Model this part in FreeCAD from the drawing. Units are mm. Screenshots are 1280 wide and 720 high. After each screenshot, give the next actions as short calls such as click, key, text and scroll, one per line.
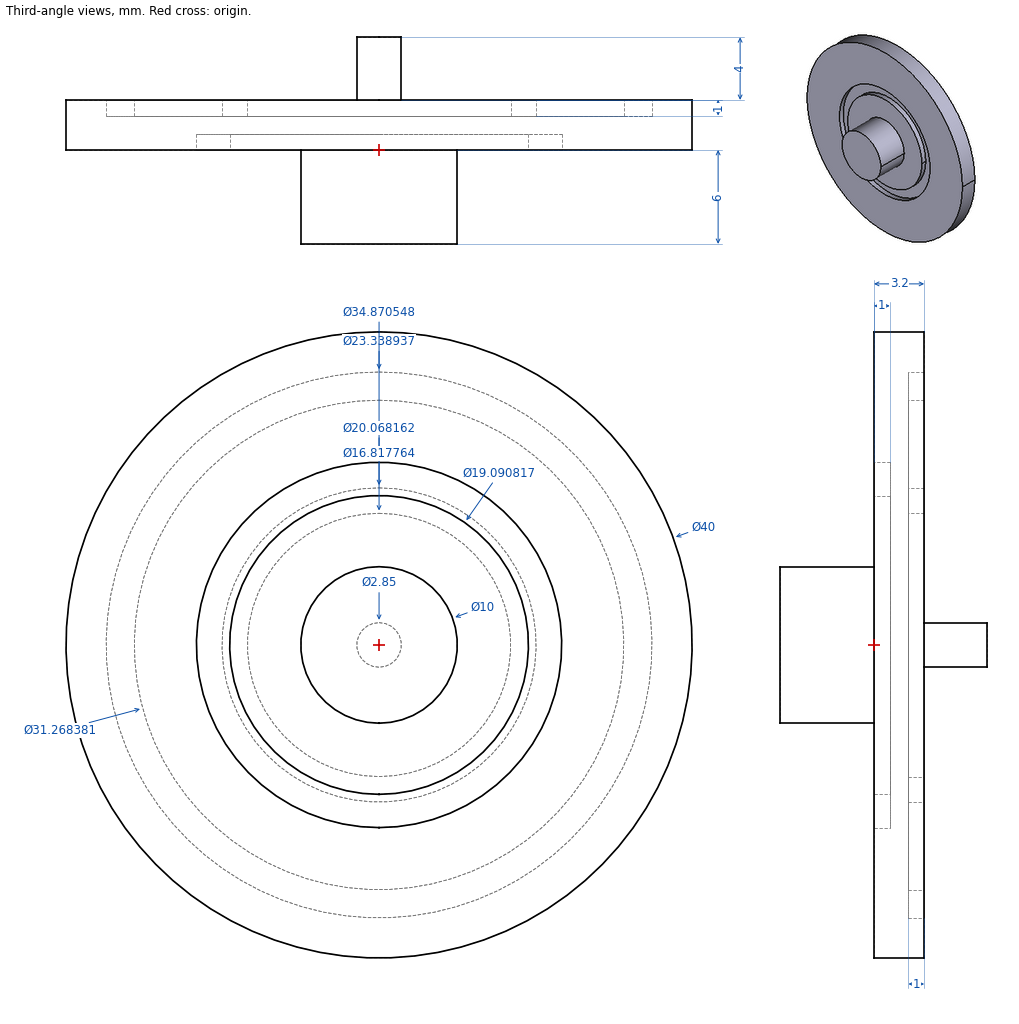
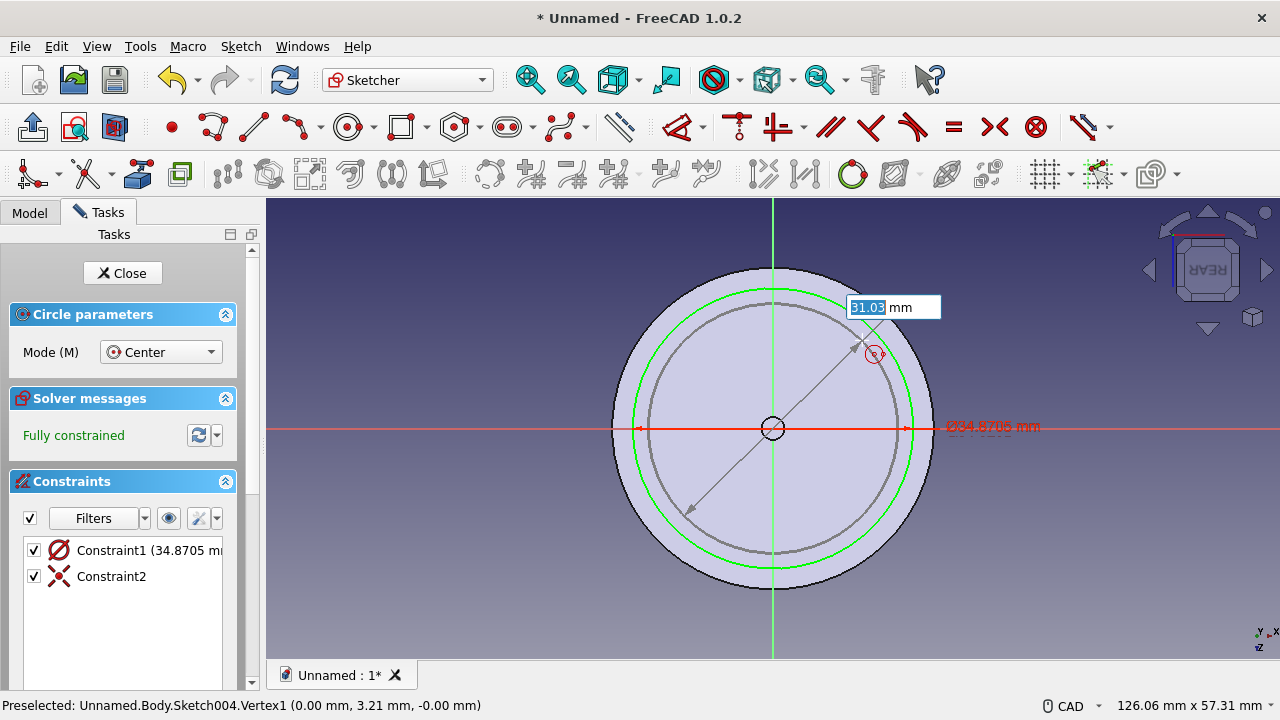
text(31.268381)
key(Return)
key(Escape)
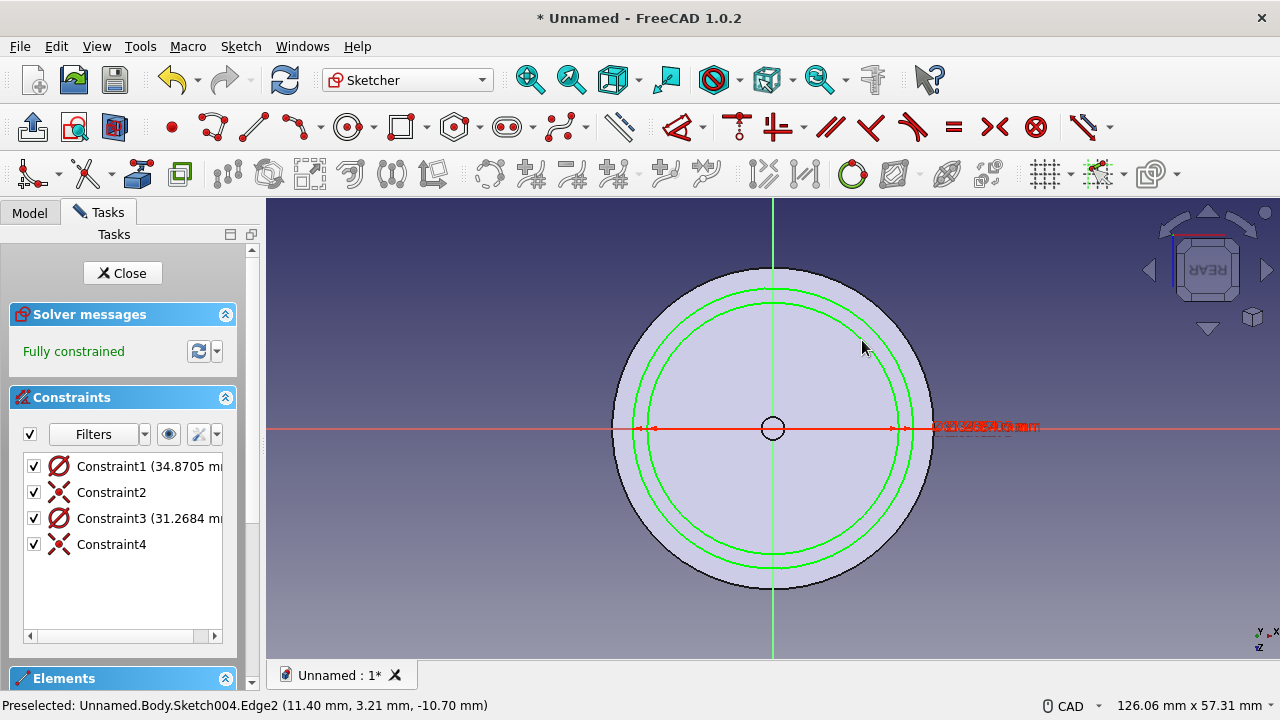
click(123, 273)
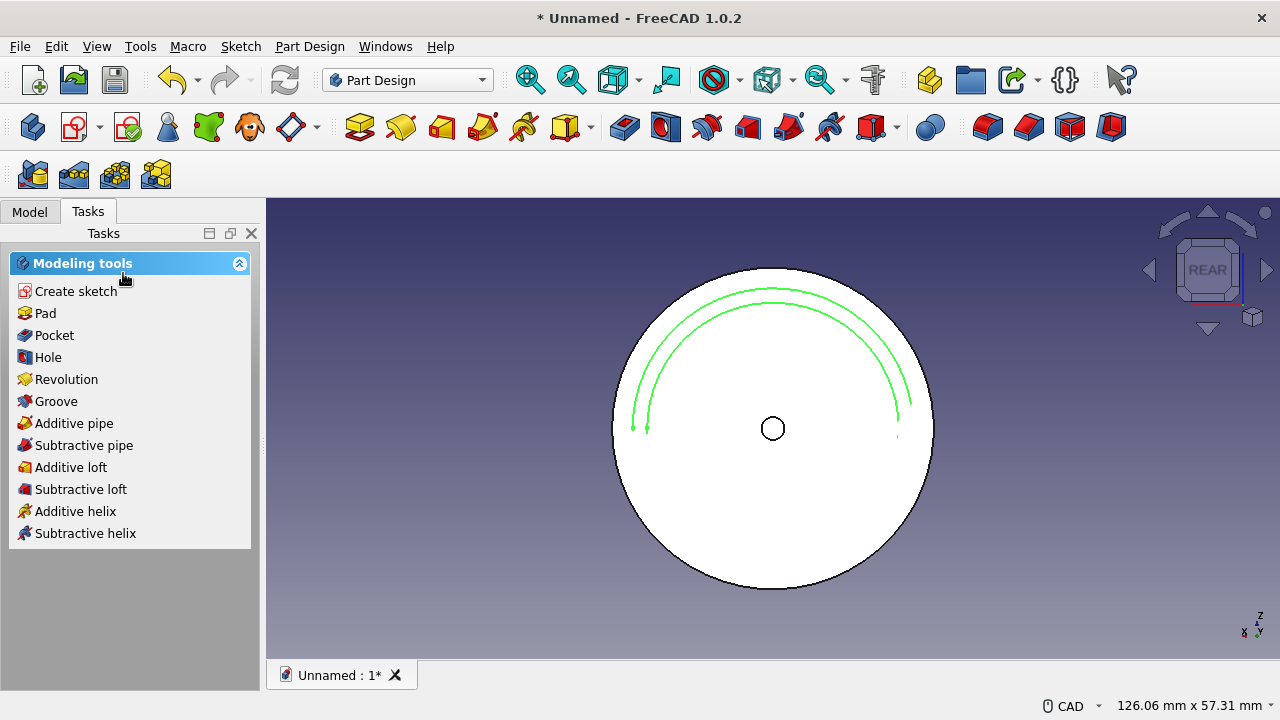
click(625, 128)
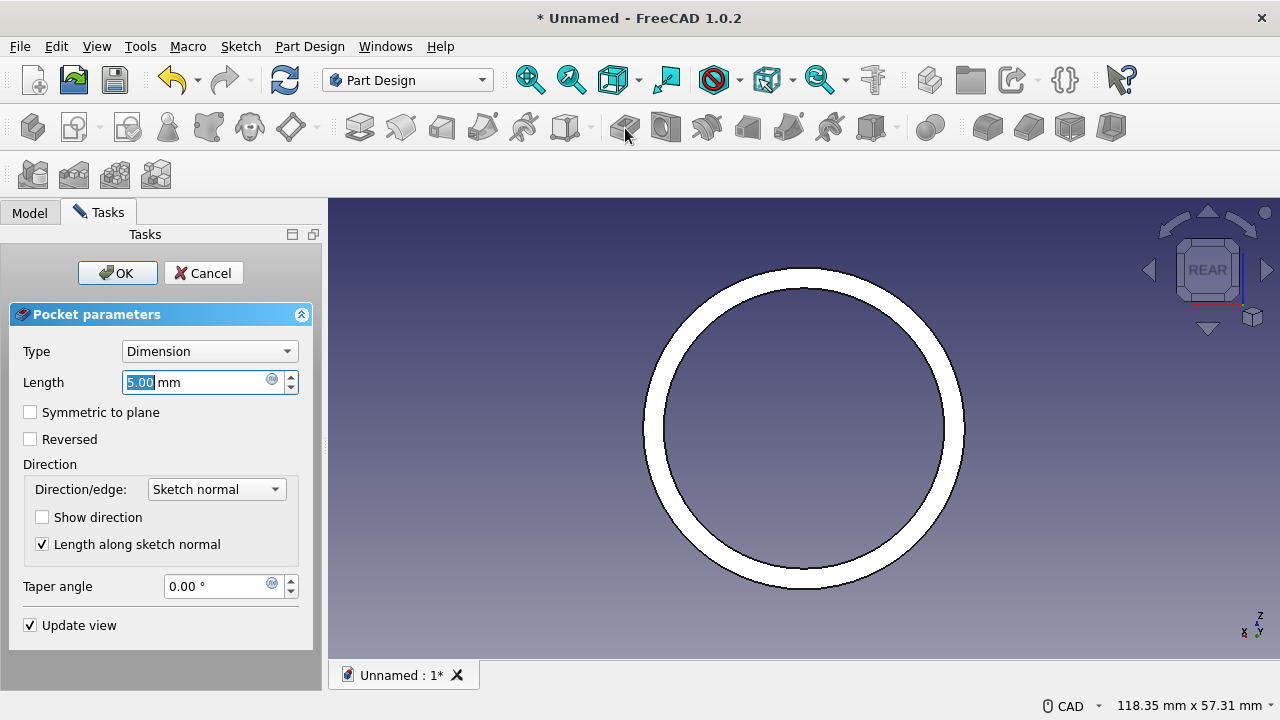
text(1)
key(Tab)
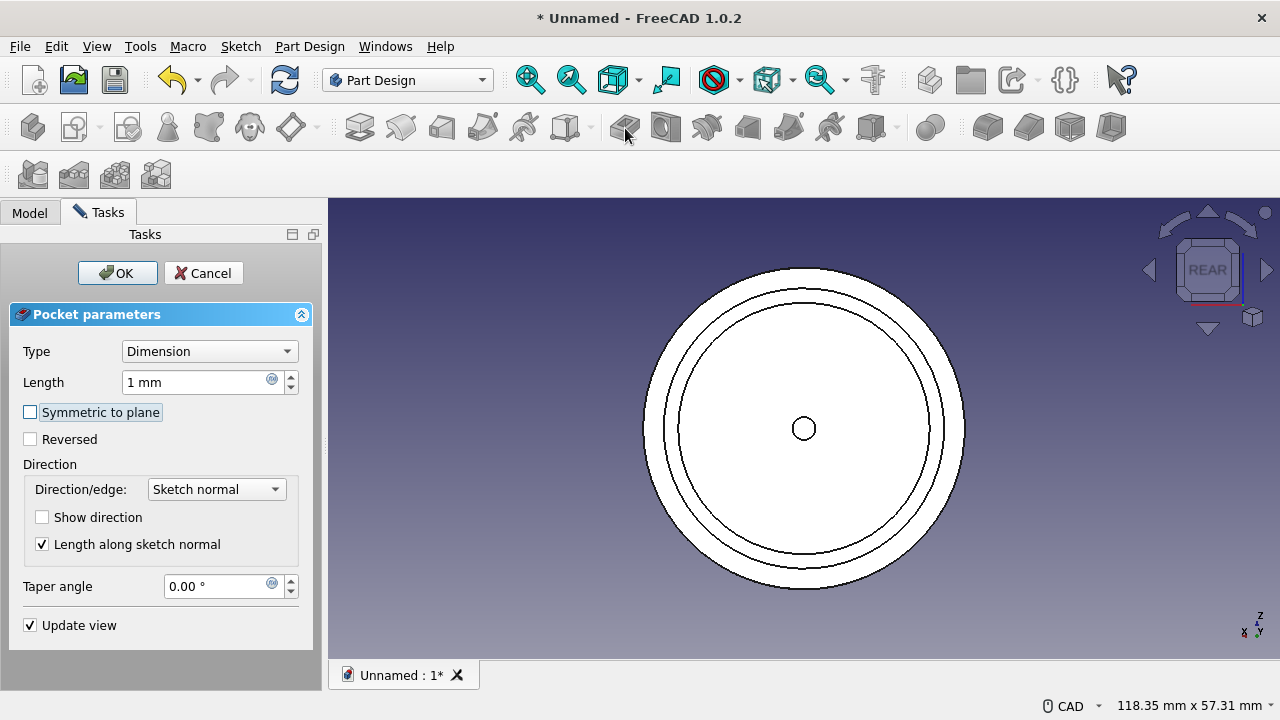
click(118, 273)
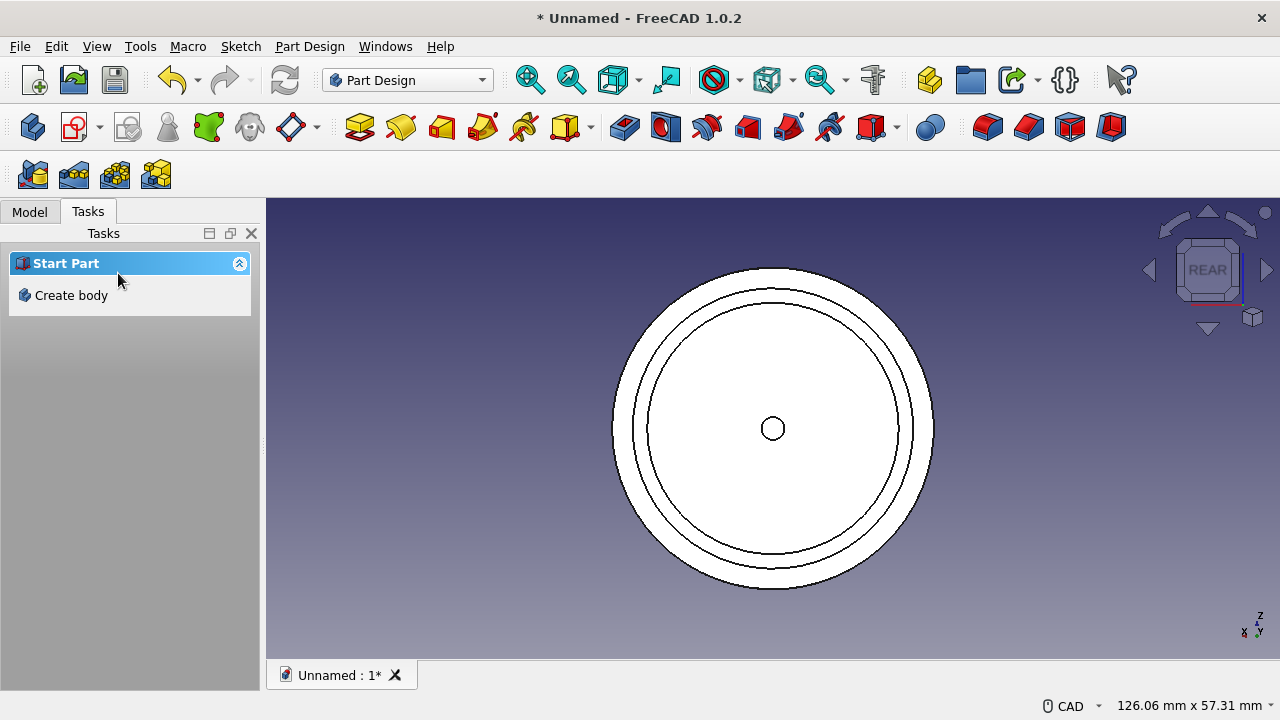
click(701, 428)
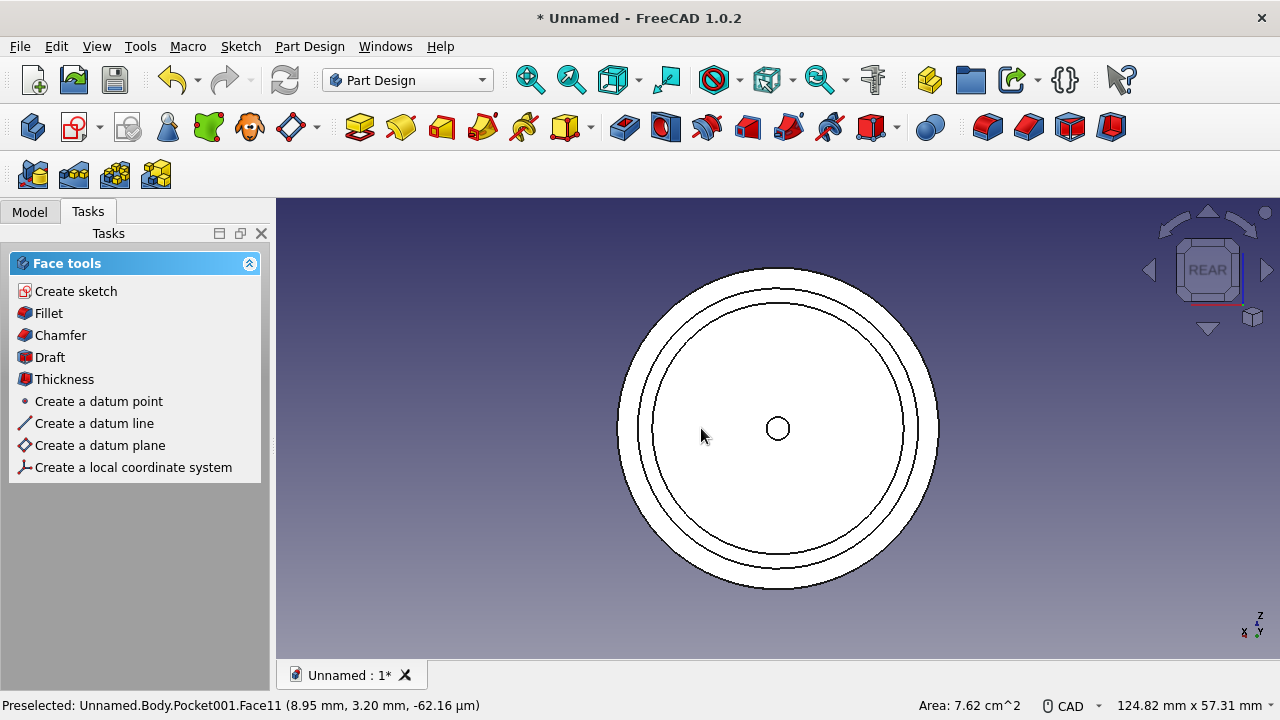
click(74, 128)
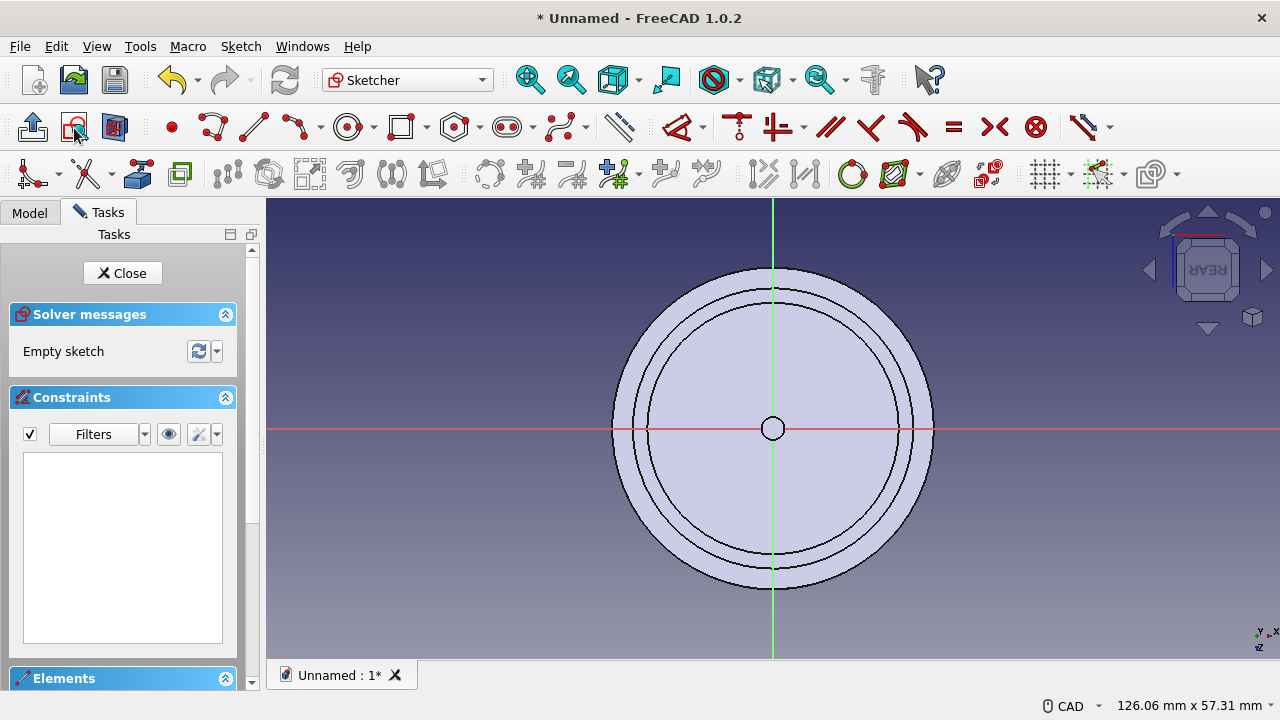
click(115, 128)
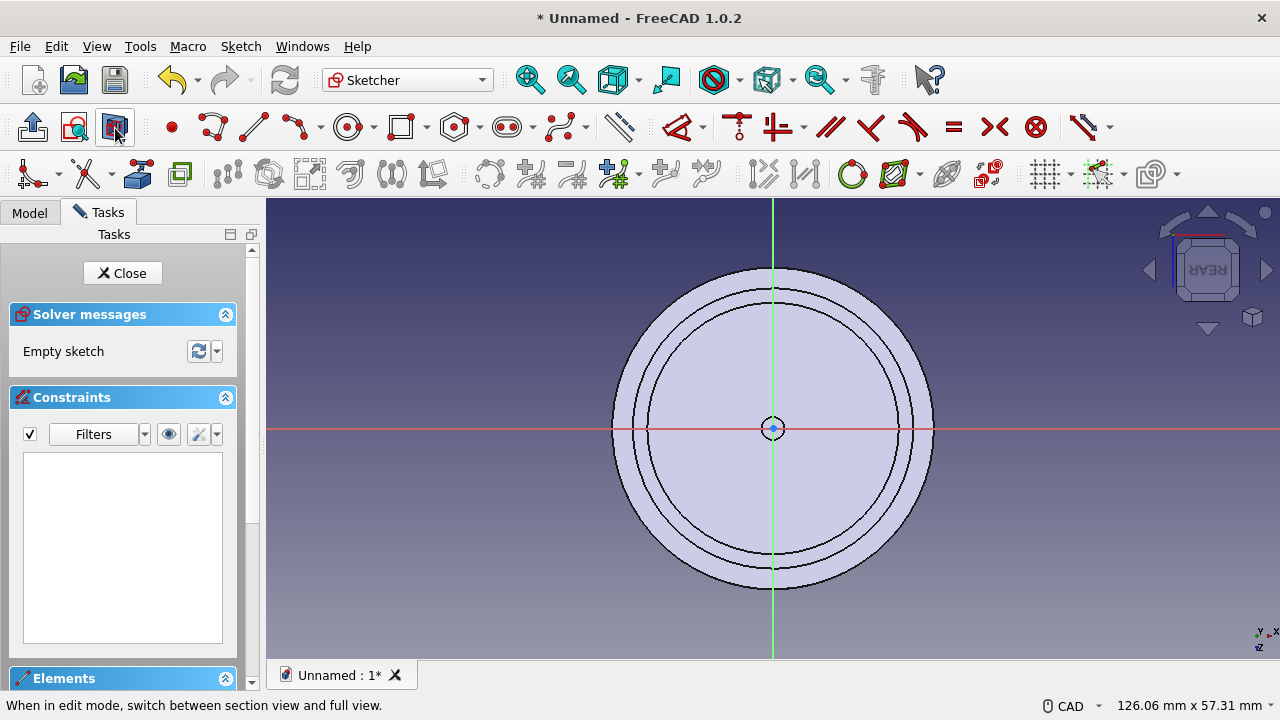
scroll(856, 428, up, 3)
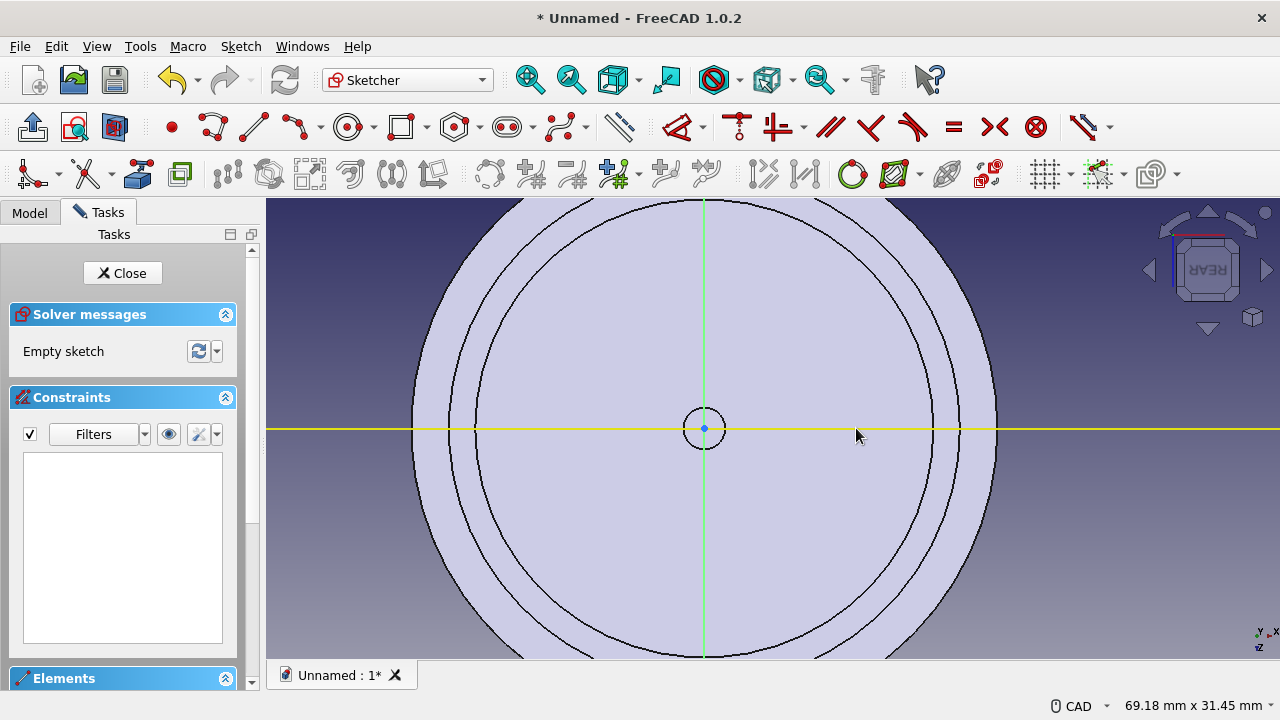
click(348, 128)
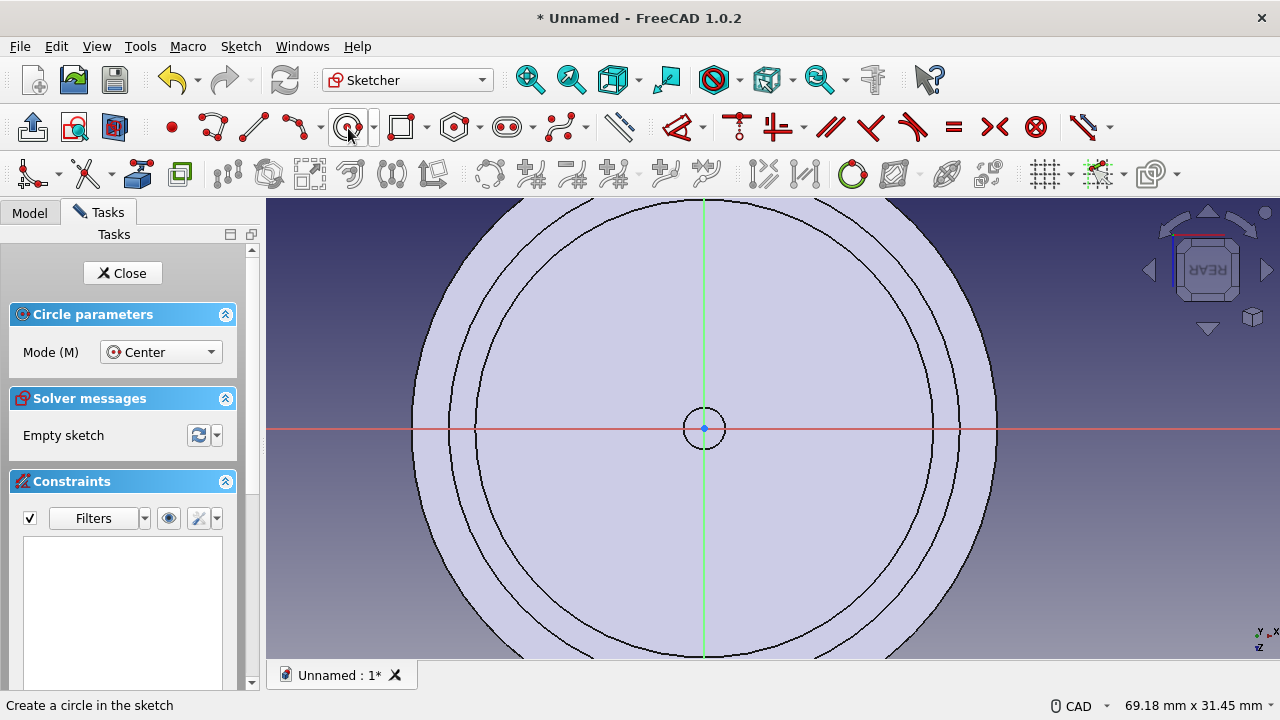
click(704, 428)
move(808, 325)